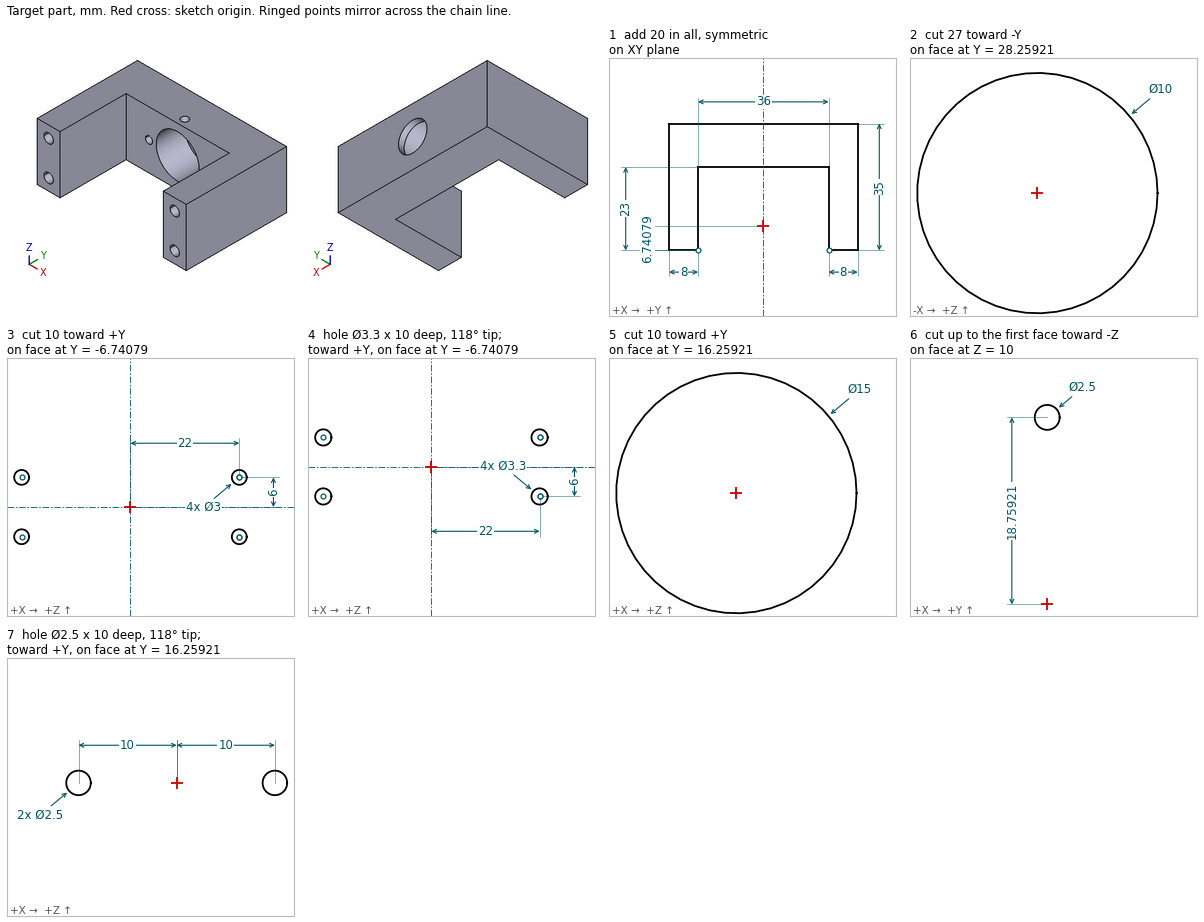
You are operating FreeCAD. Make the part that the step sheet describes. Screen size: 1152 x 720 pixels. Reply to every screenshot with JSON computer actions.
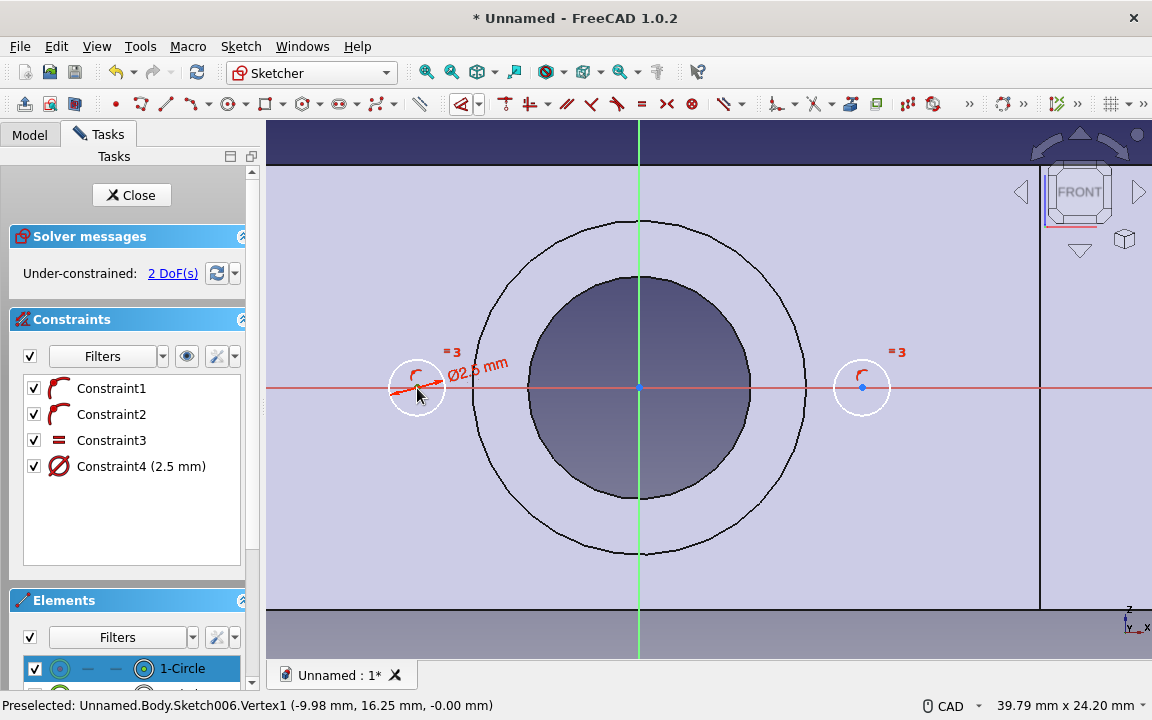
{"action": "key", "text": "l"}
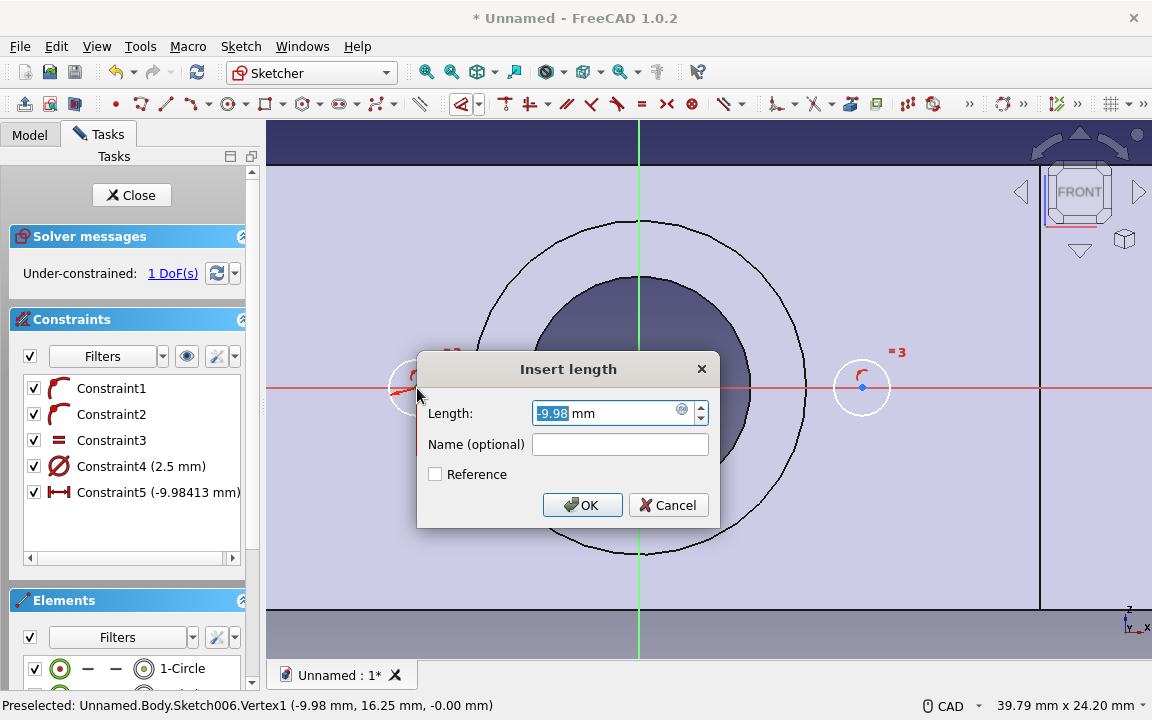
{"action": "type", "text": "-10"}
{"action": "key", "text": "Return"}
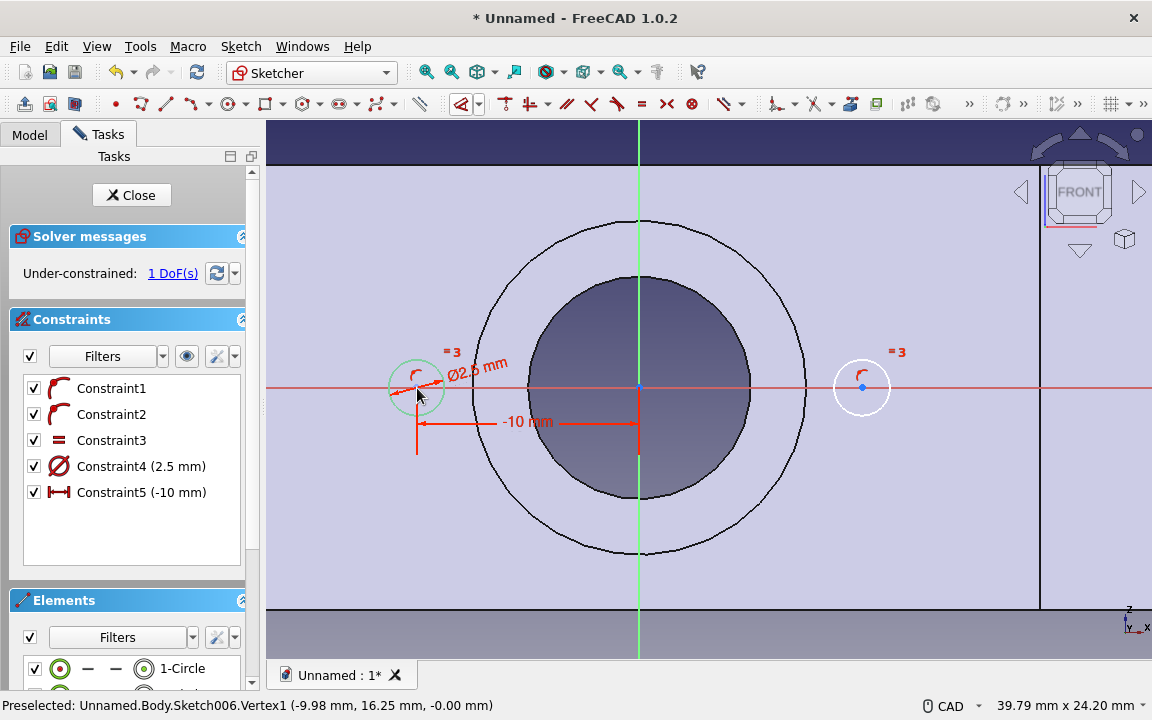
{"action": "left_click", "coordinate": [862, 388]}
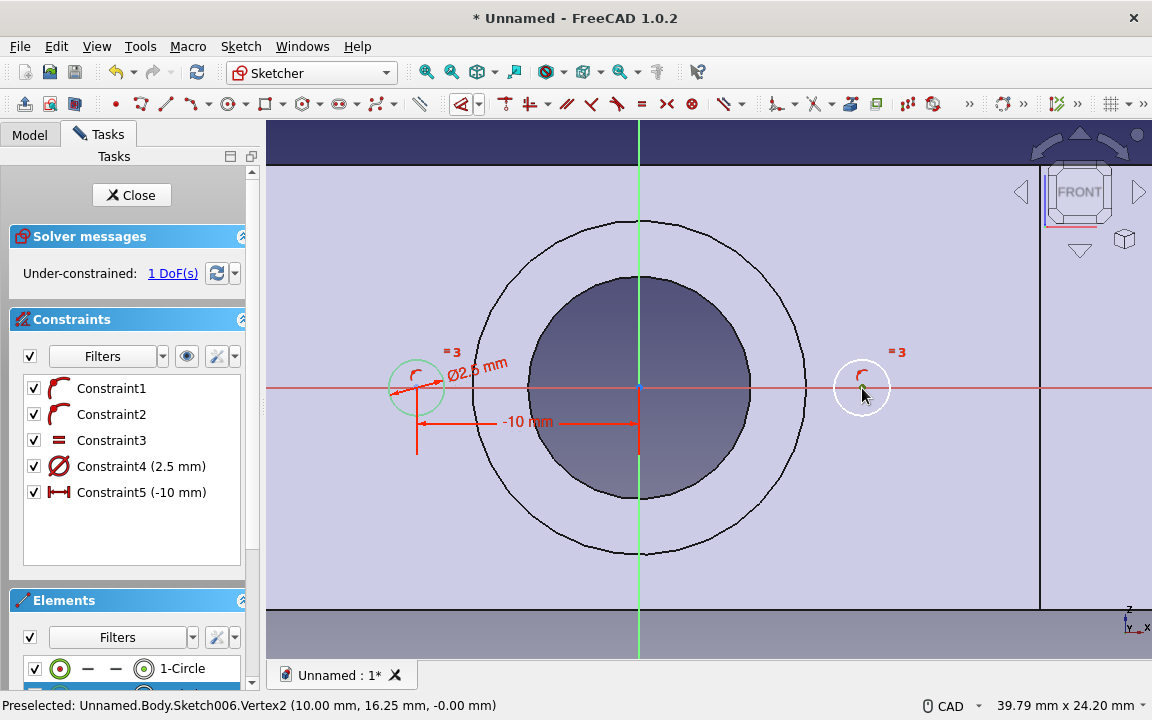
{"action": "key", "text": "l"}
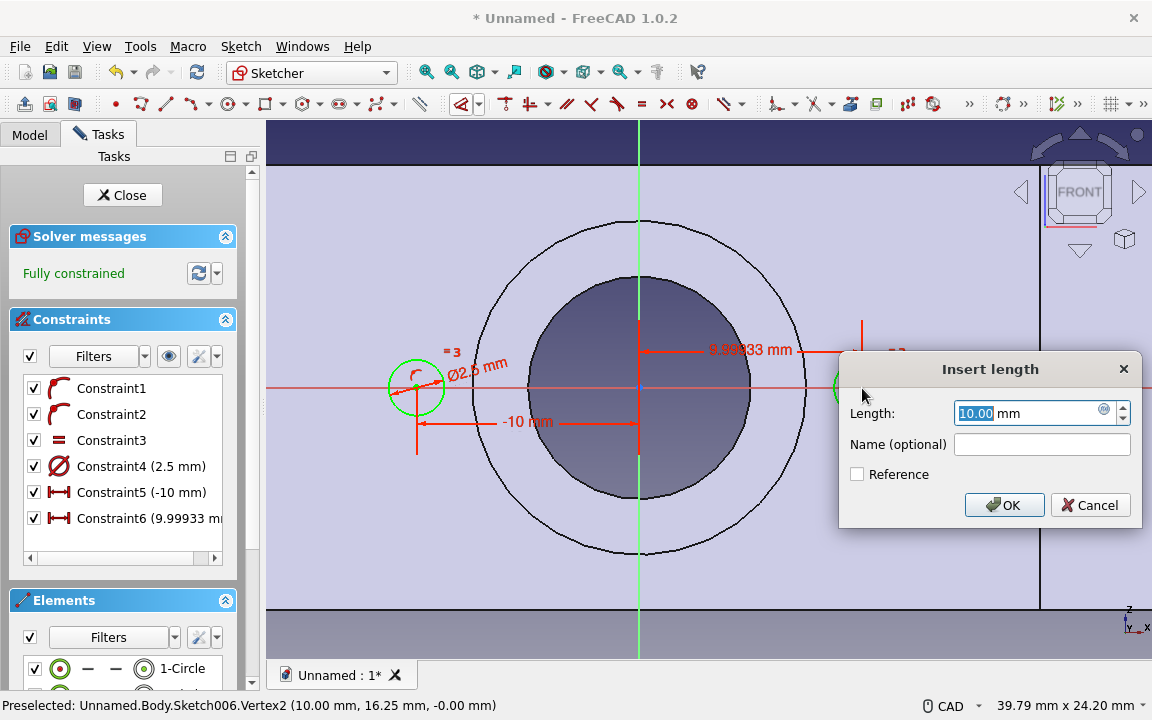
{"action": "type", "text": "10"}
{"action": "key", "text": "Return"}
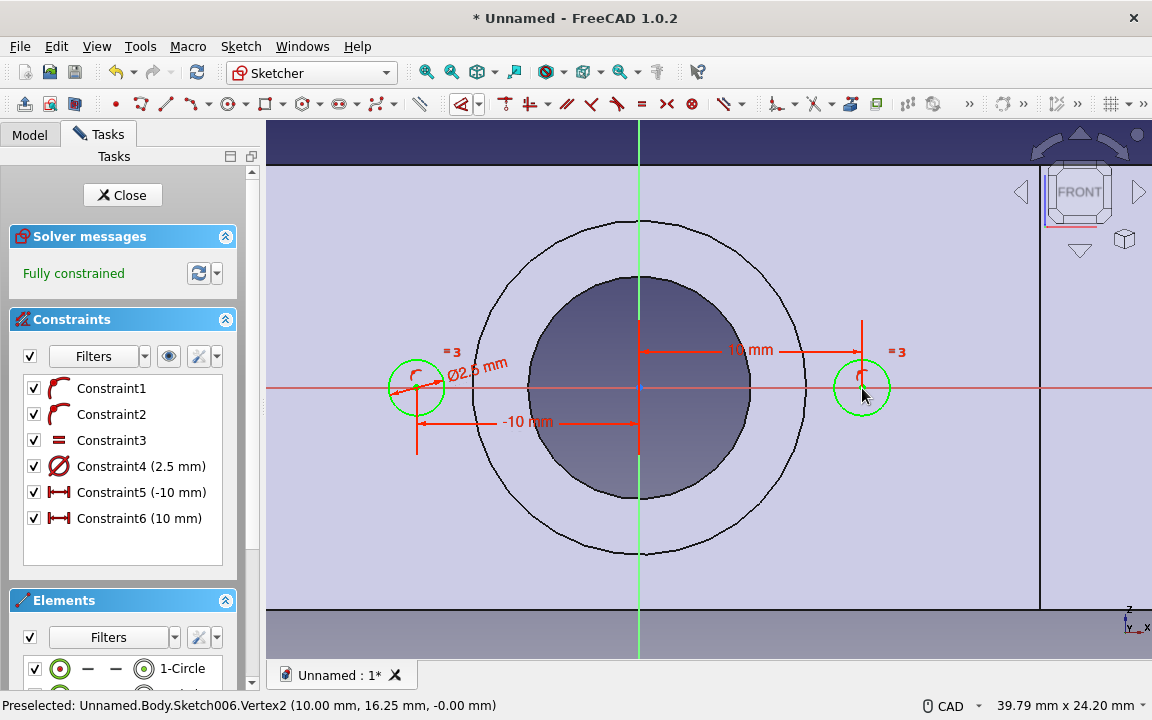
{"action": "left_click", "coordinate": [123, 195]}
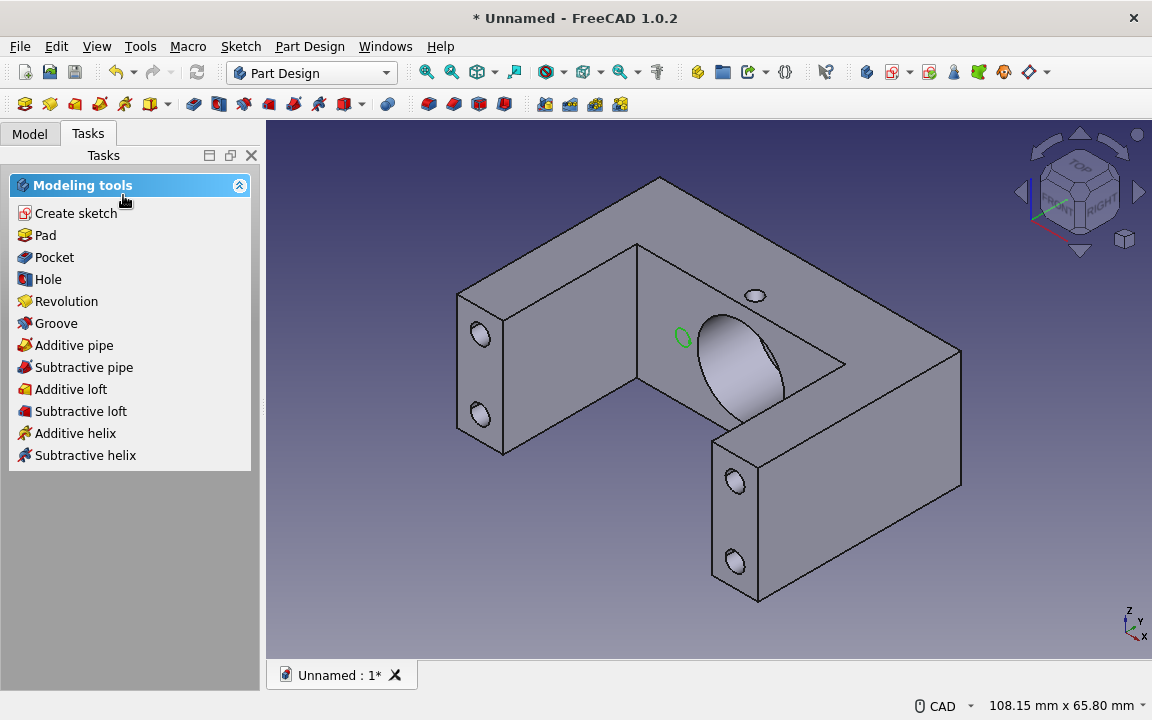
{"action": "left_click", "coordinate": [219, 104]}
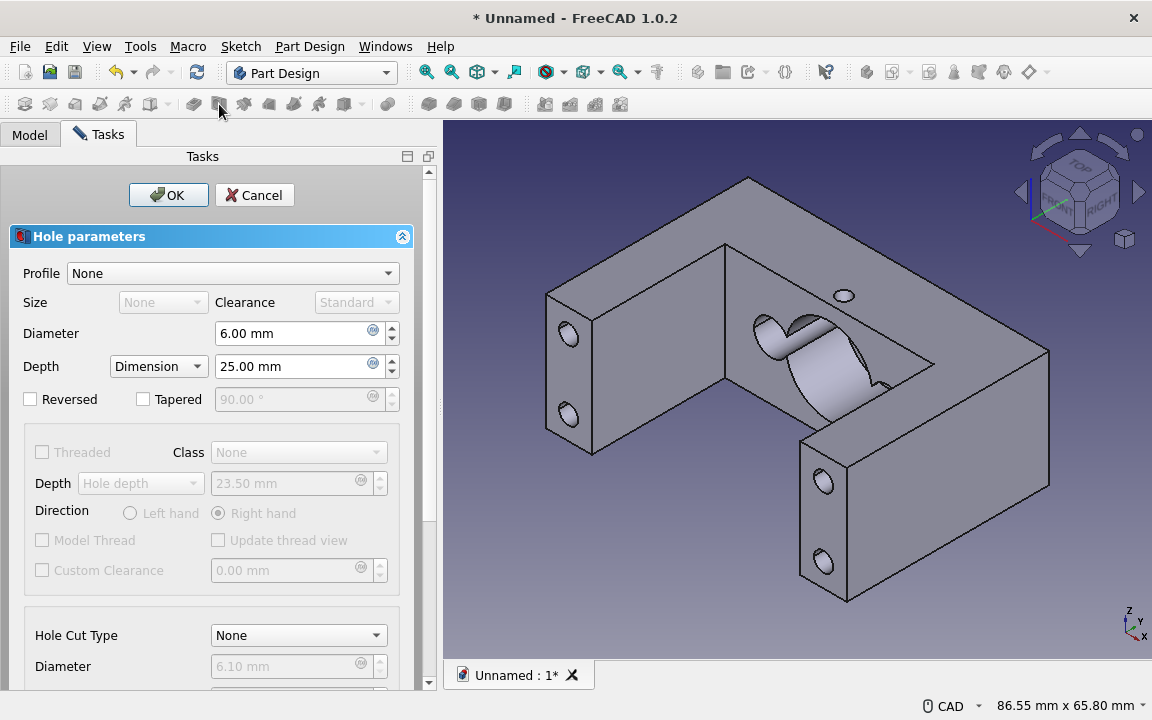
{"action": "triple_click", "coordinate": [300, 334]}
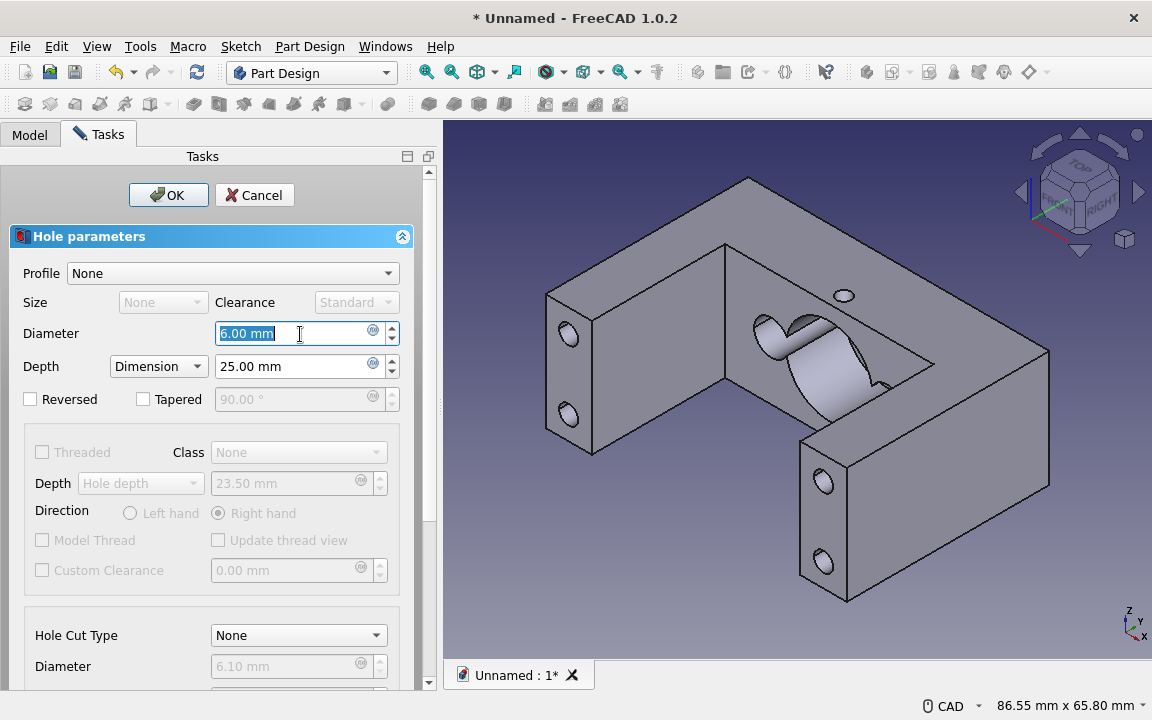
{"action": "type", "text": "2.5"}
{"action": "key", "text": "Tab"}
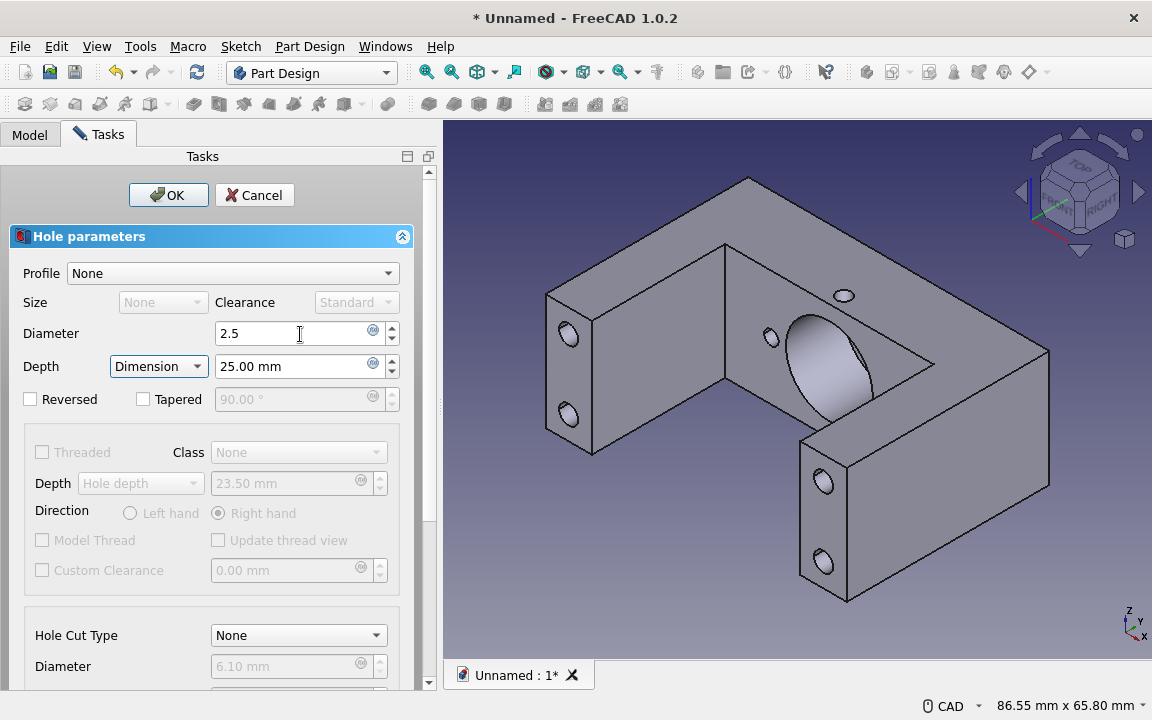
{"action": "triple_click", "coordinate": [300, 366]}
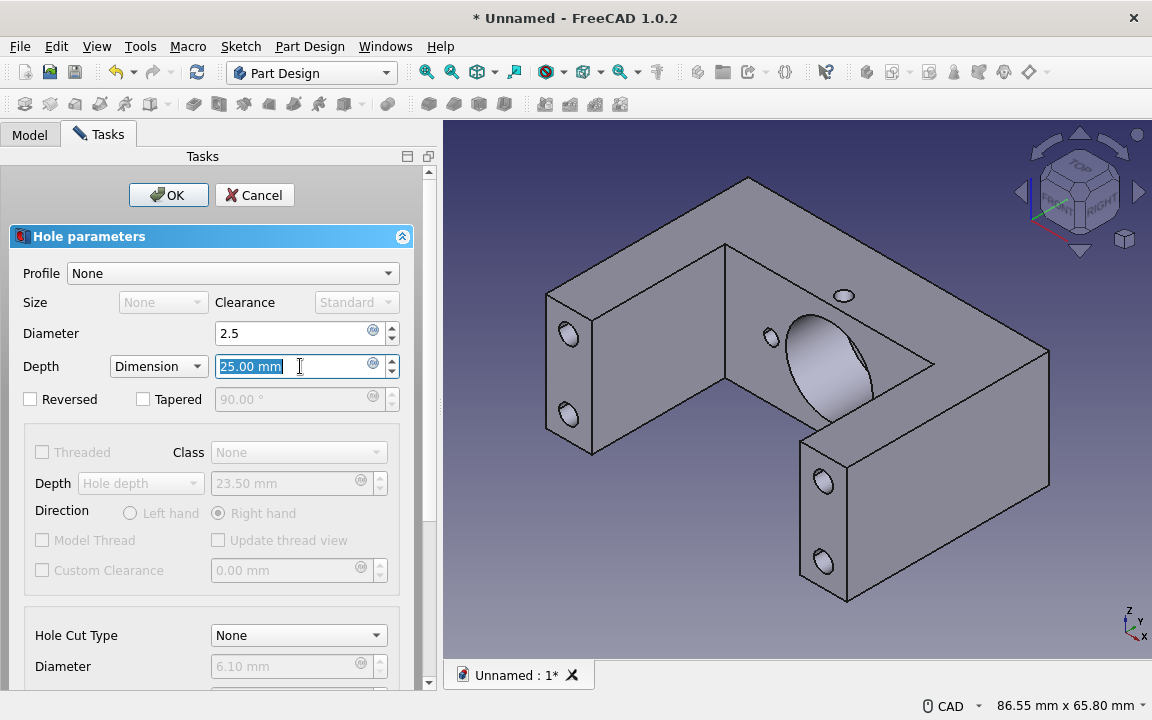
{"action": "type", "text": "10"}
{"action": "key", "text": "Tab"}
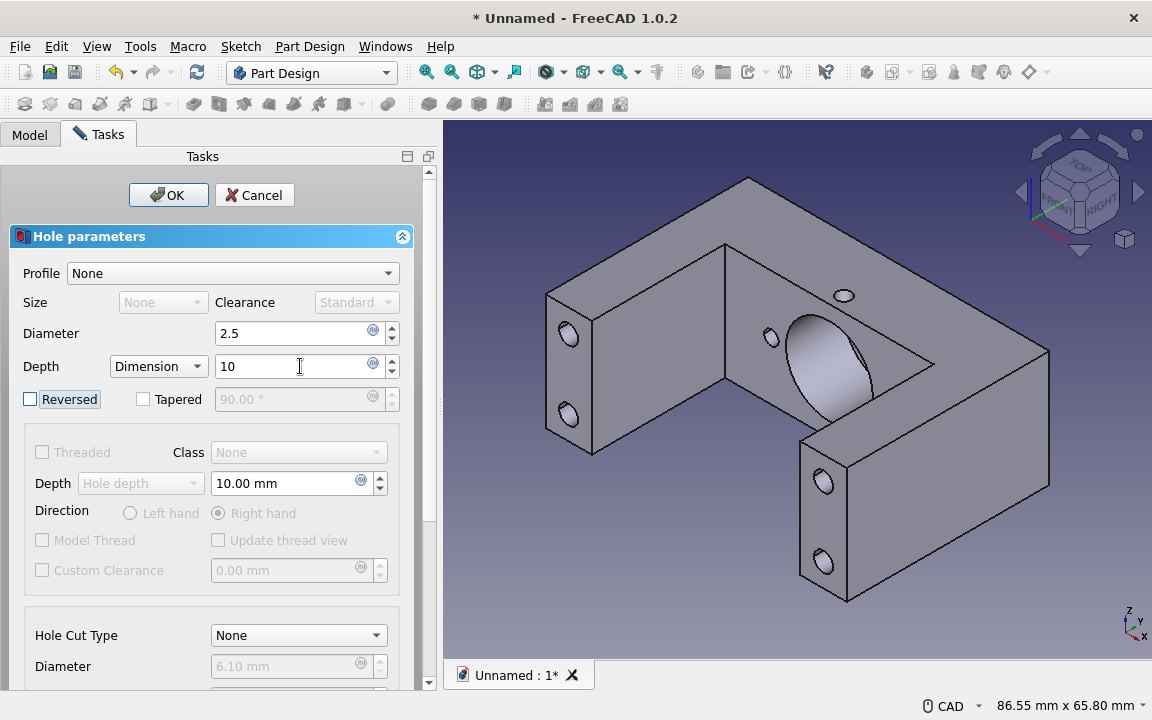
{"action": "left_click", "coordinate": [169, 195]}